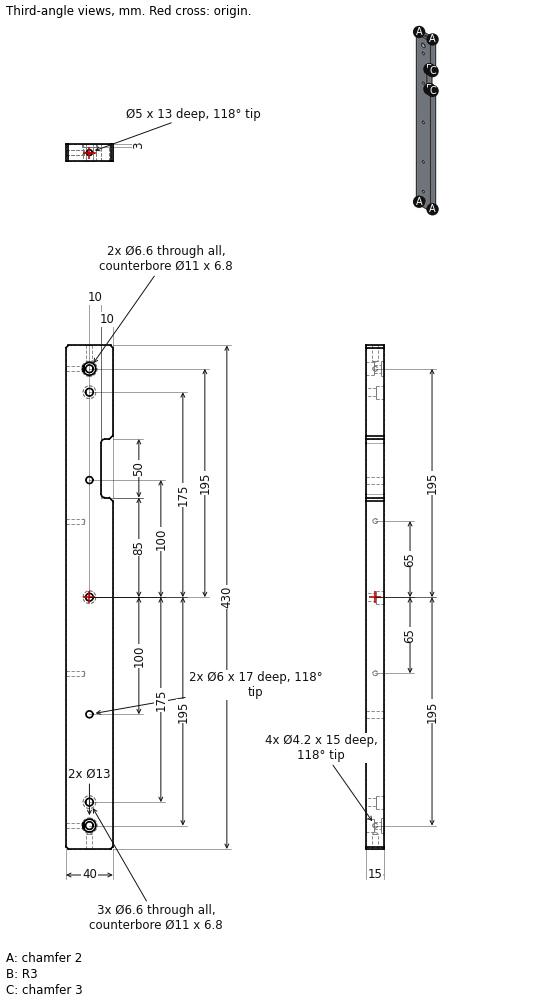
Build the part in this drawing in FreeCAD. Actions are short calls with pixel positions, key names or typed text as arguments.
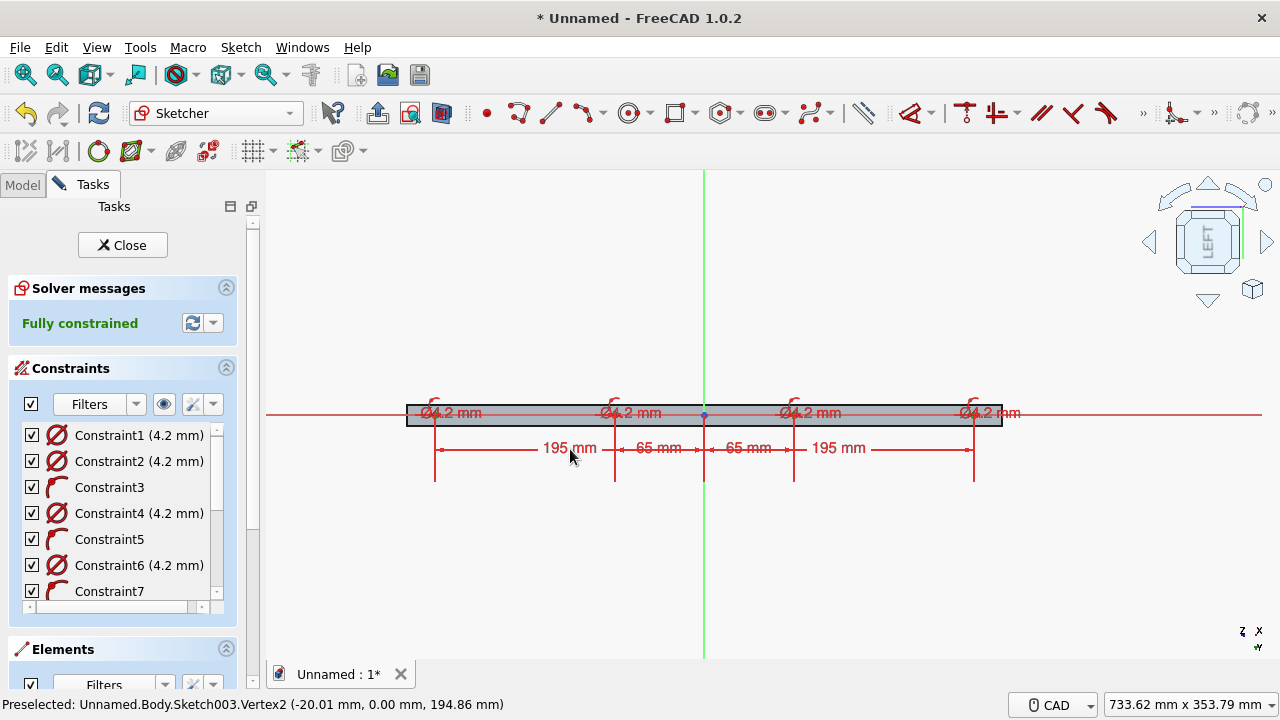
click(123, 245)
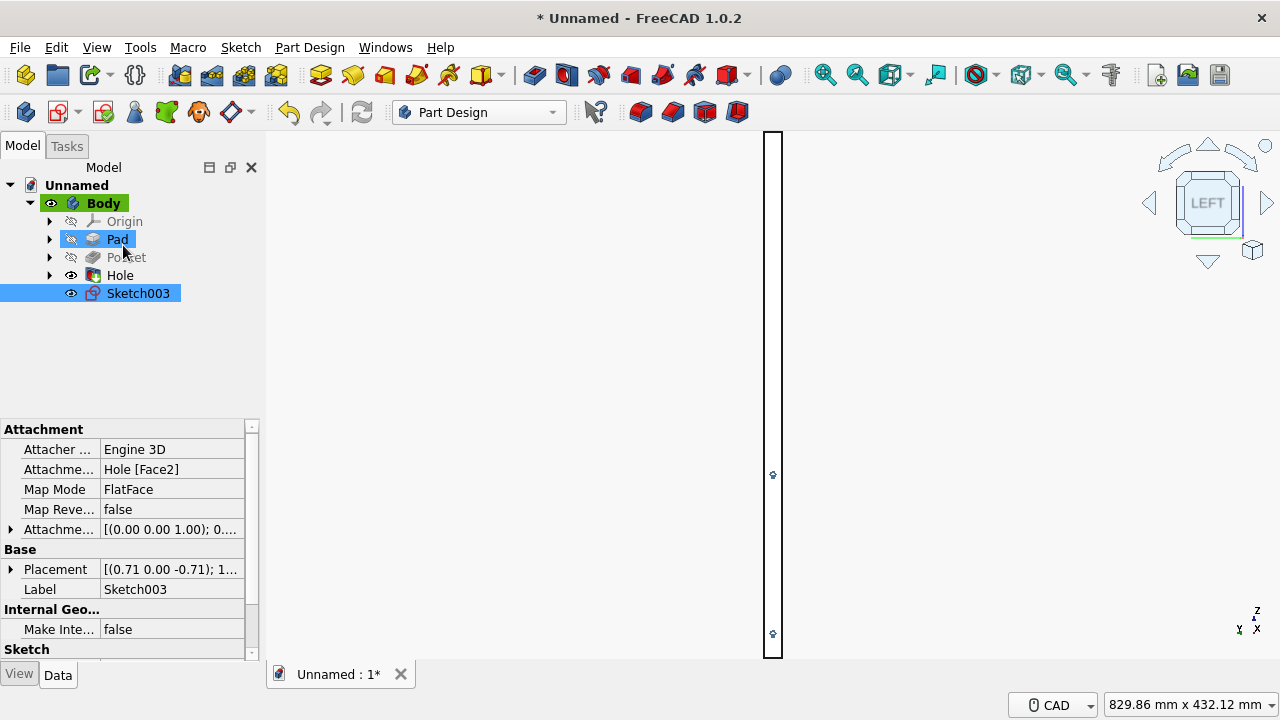
click(568, 76)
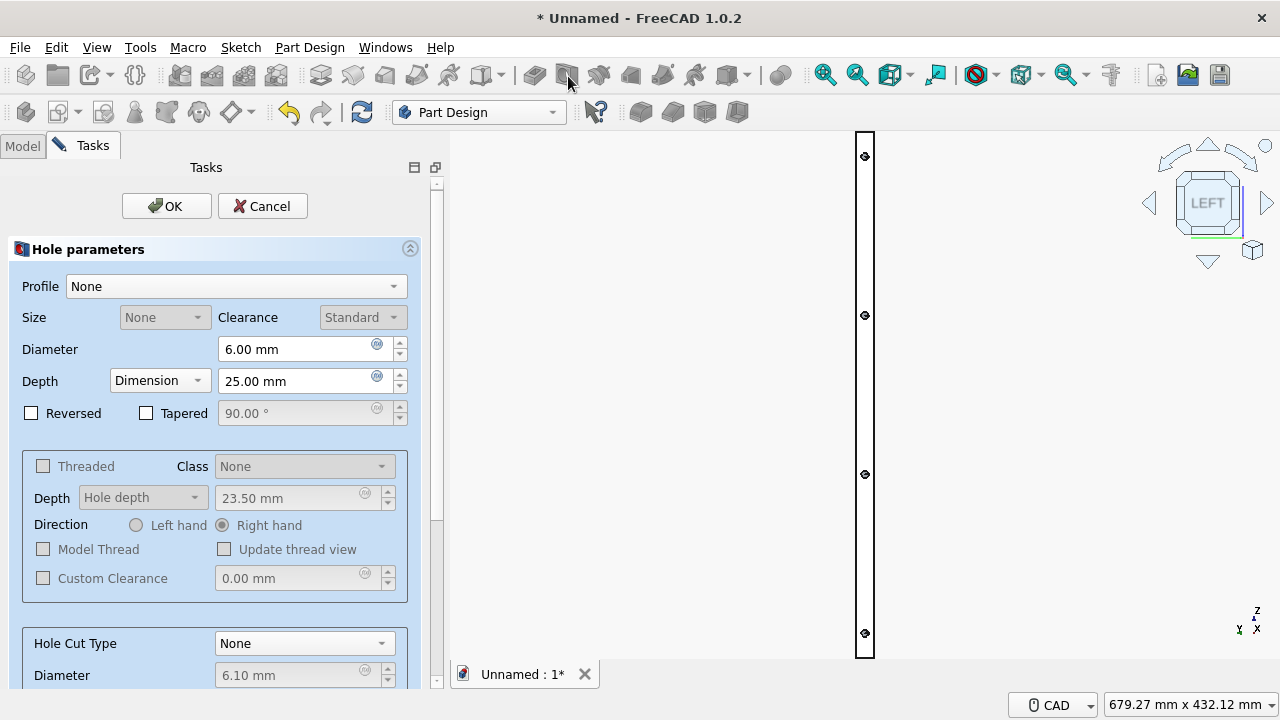
triple_click(305, 349)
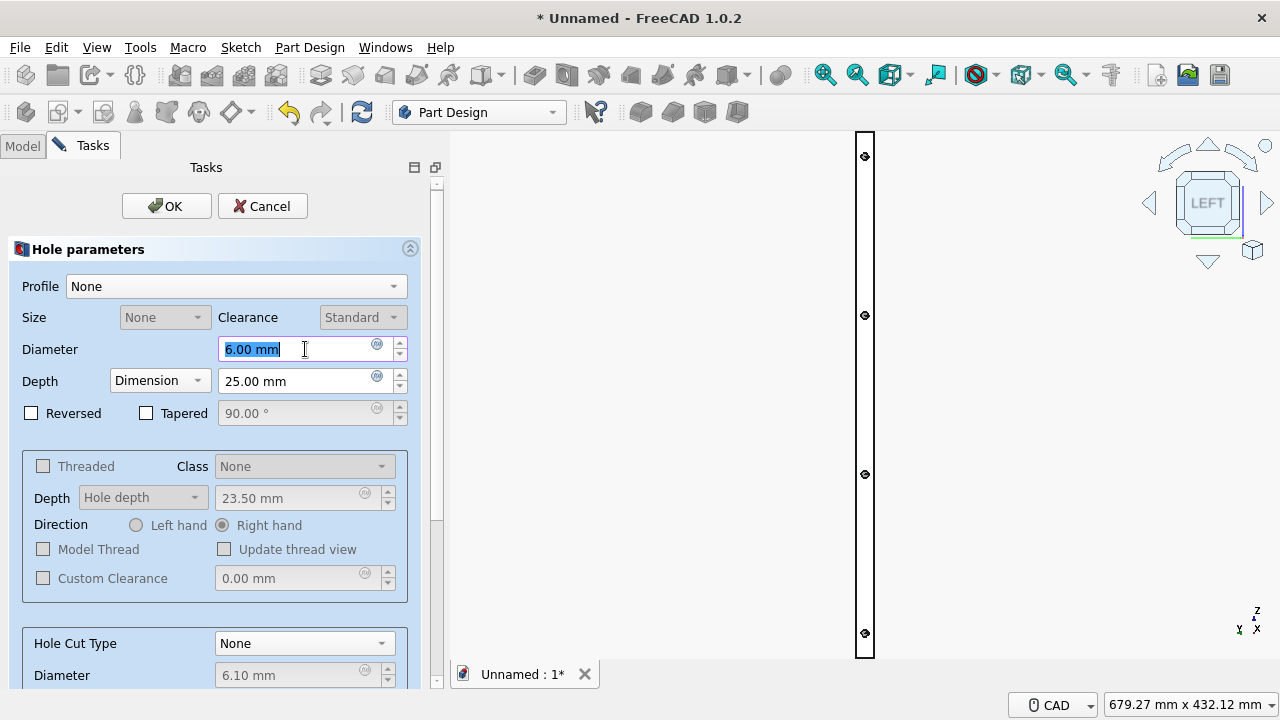
text(4.2)
key(Tab)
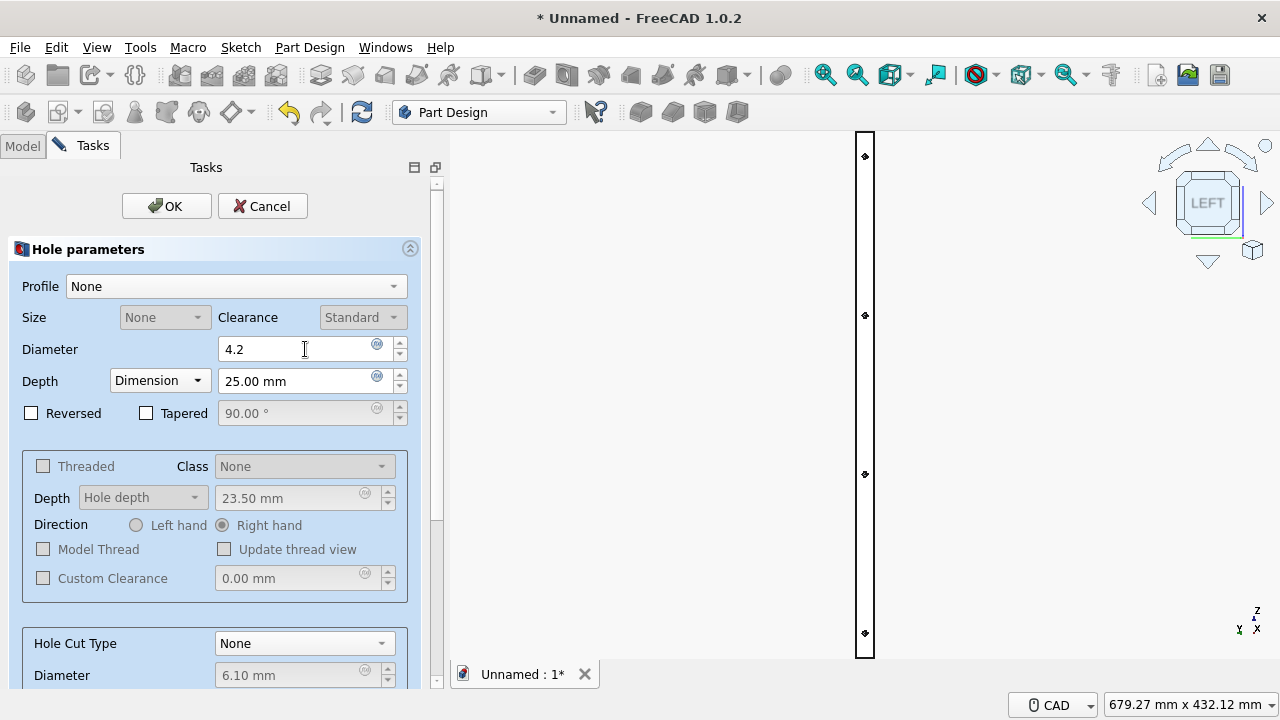
triple_click(305, 381)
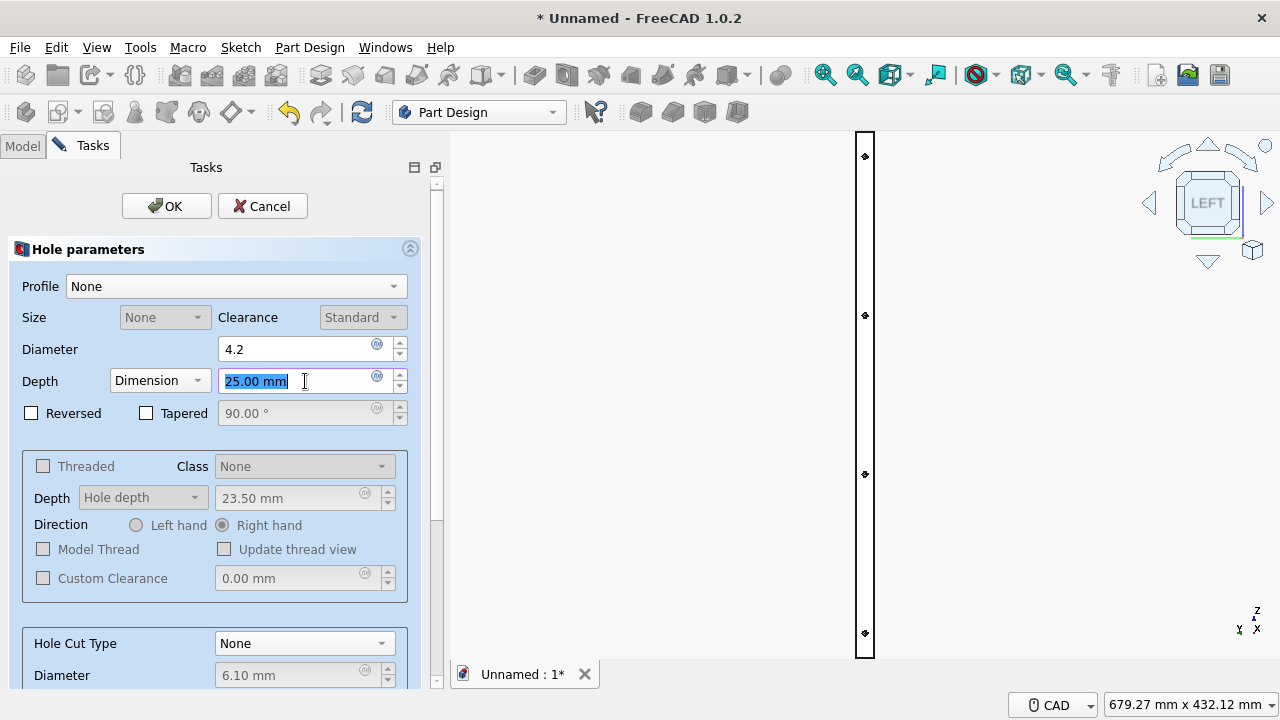
text(15)
key(Tab)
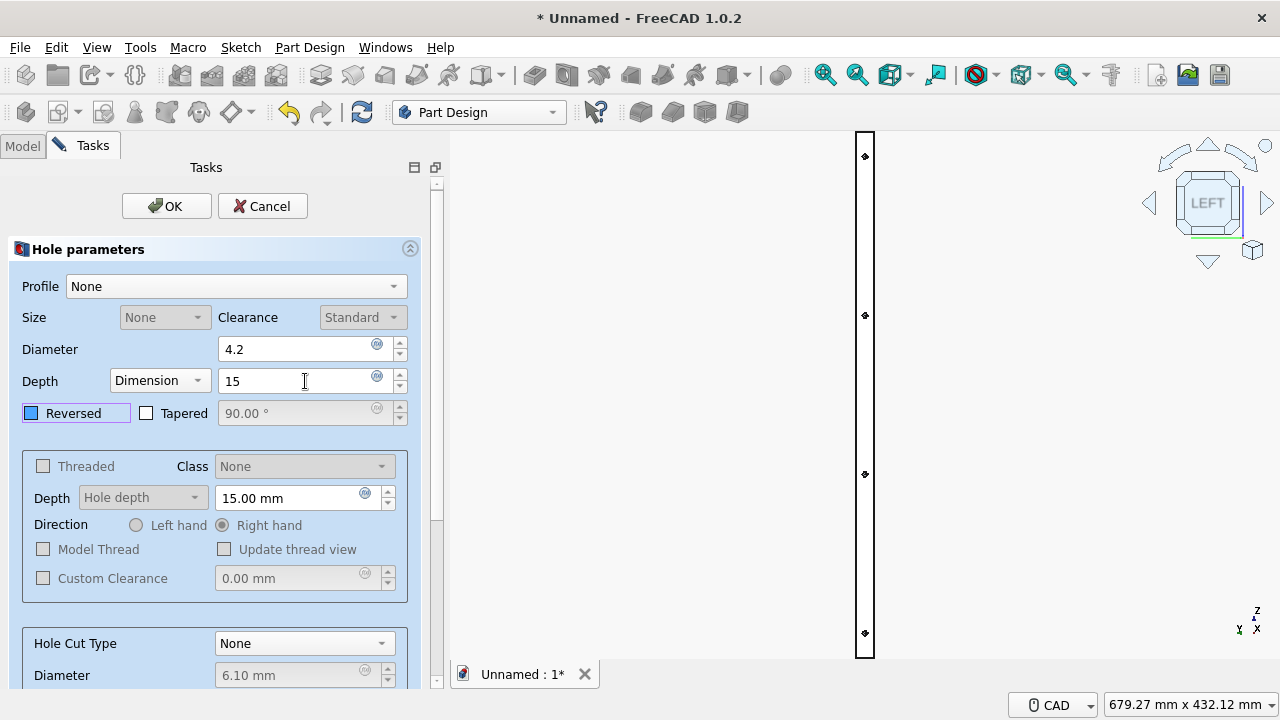
click(167, 206)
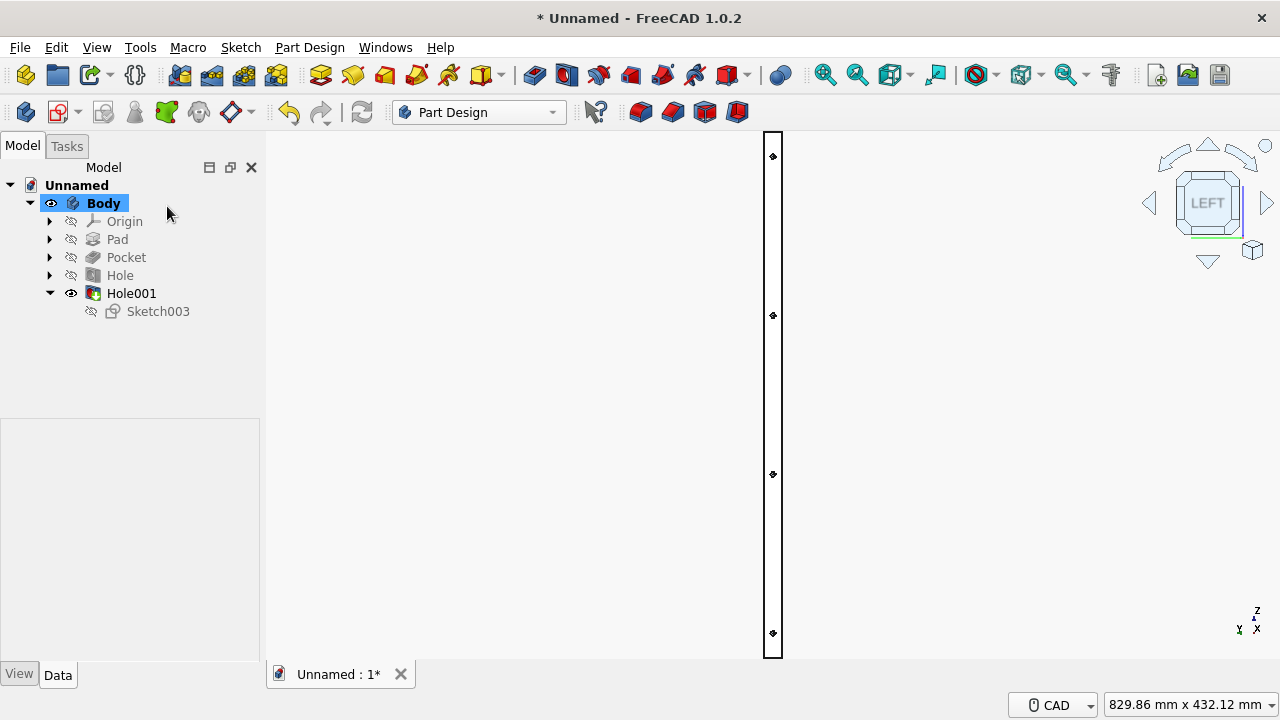
key(0)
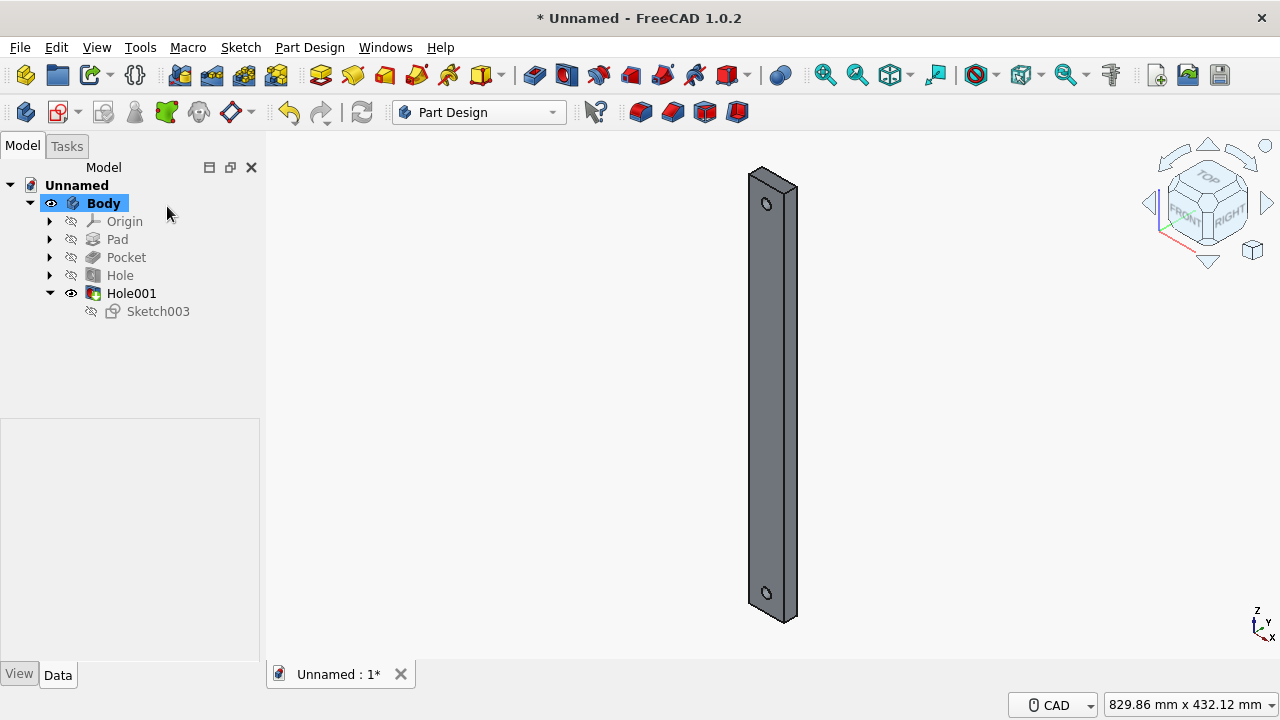
click(790, 189)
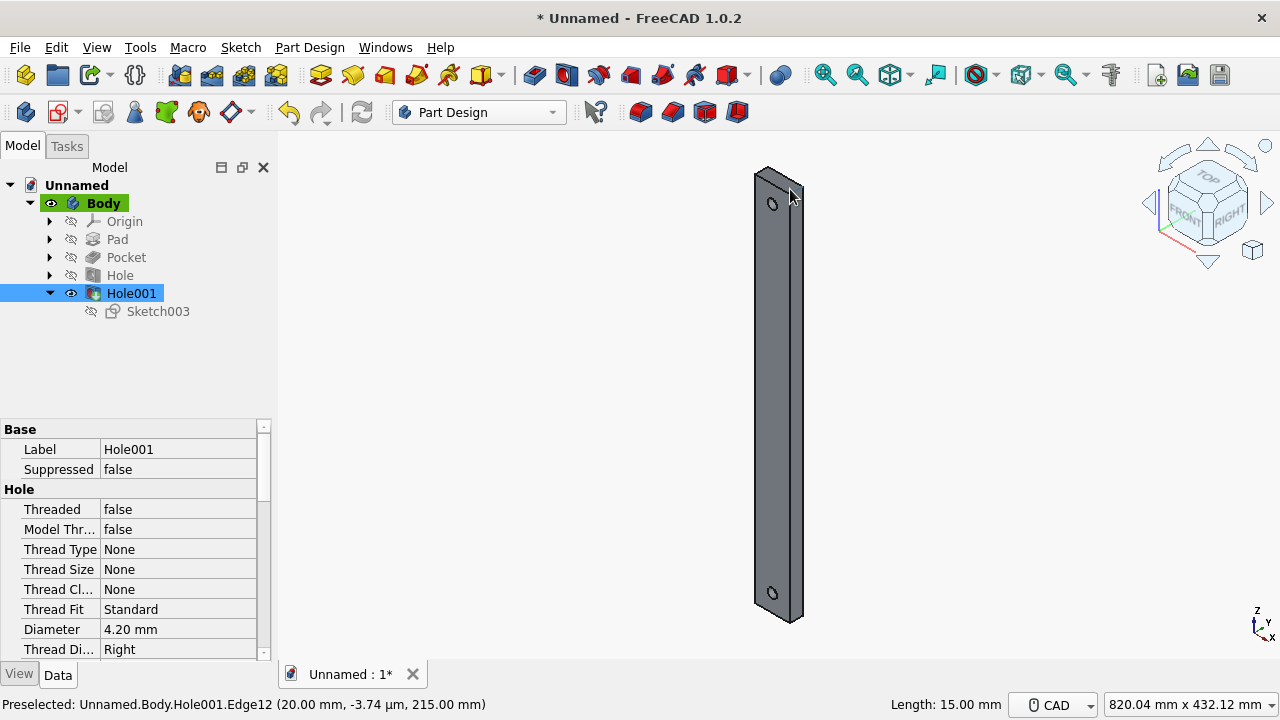
scroll(762, 599, up, 4)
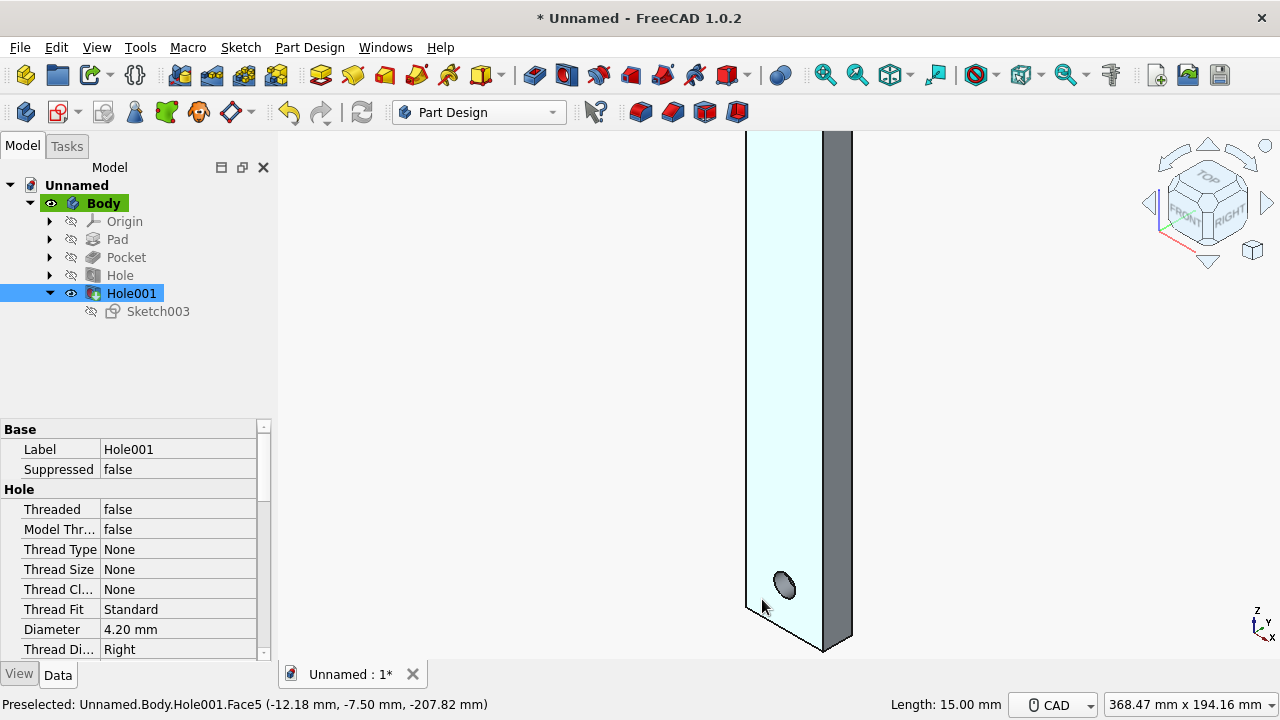
click(826, 76)